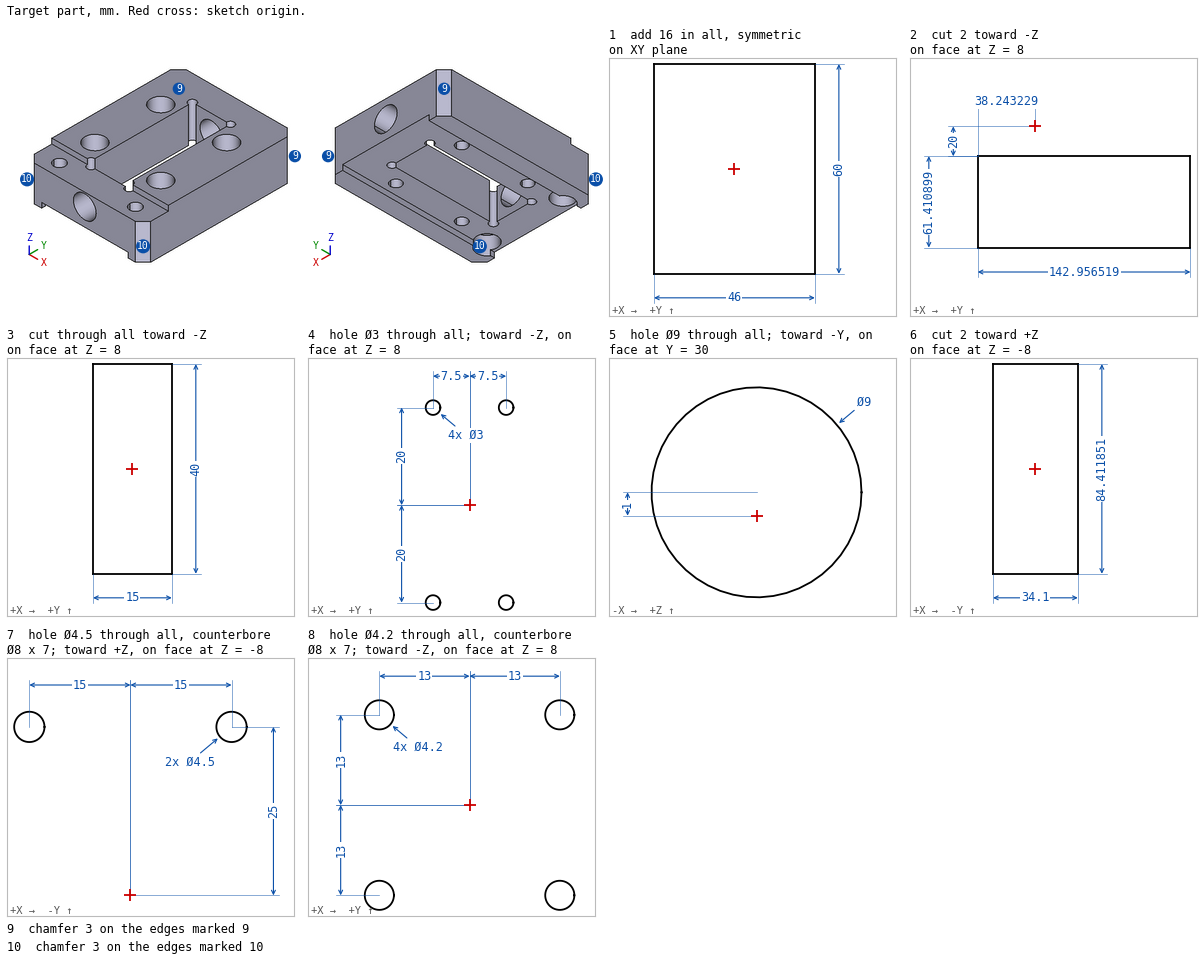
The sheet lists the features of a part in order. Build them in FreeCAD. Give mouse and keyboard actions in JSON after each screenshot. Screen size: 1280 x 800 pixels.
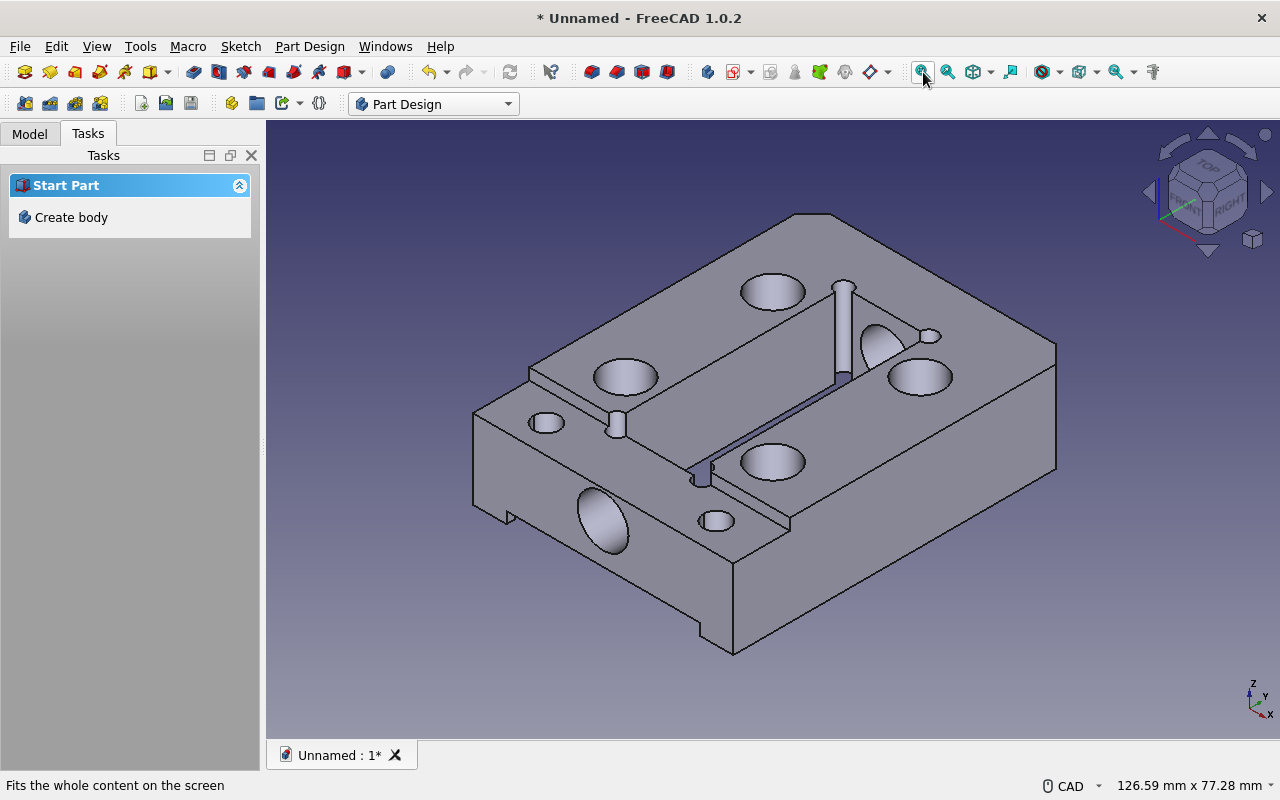
{"action": "left_click", "coordinate": [733, 608]}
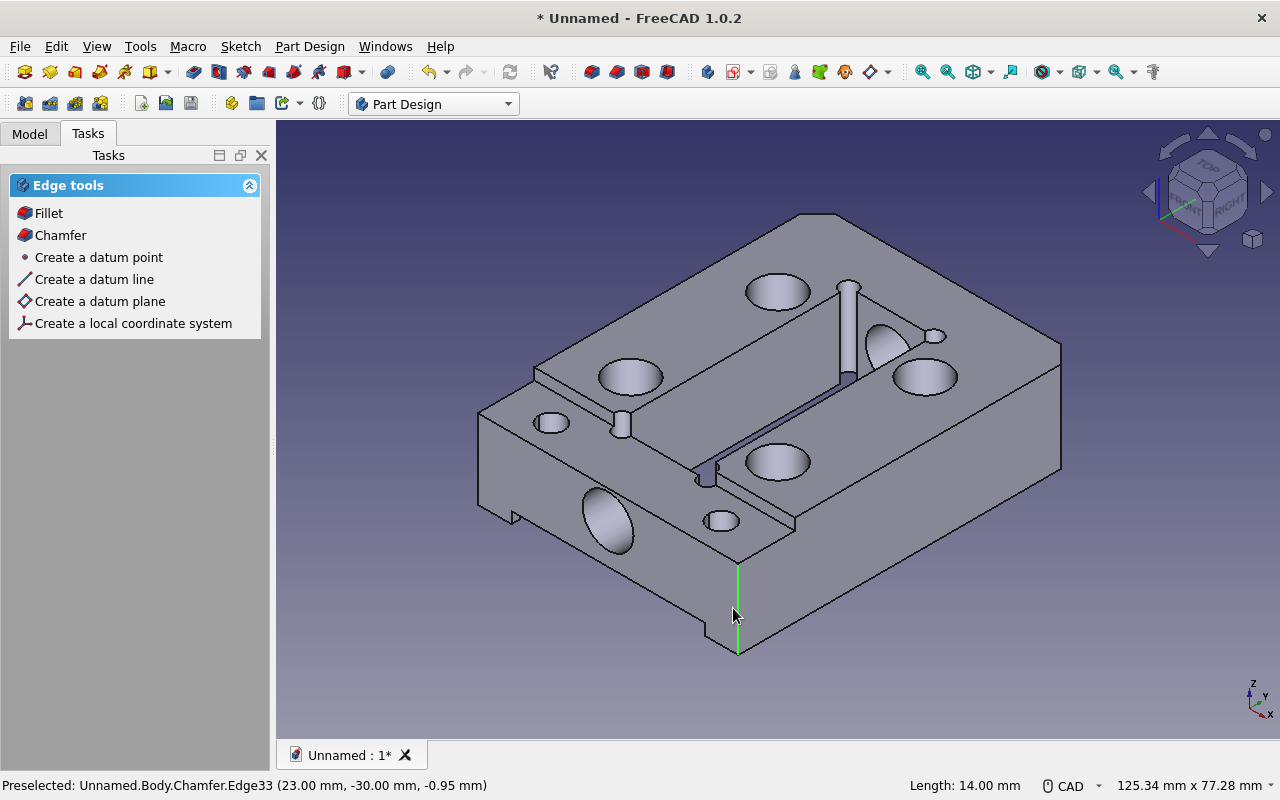
{"action": "key", "text": "2"}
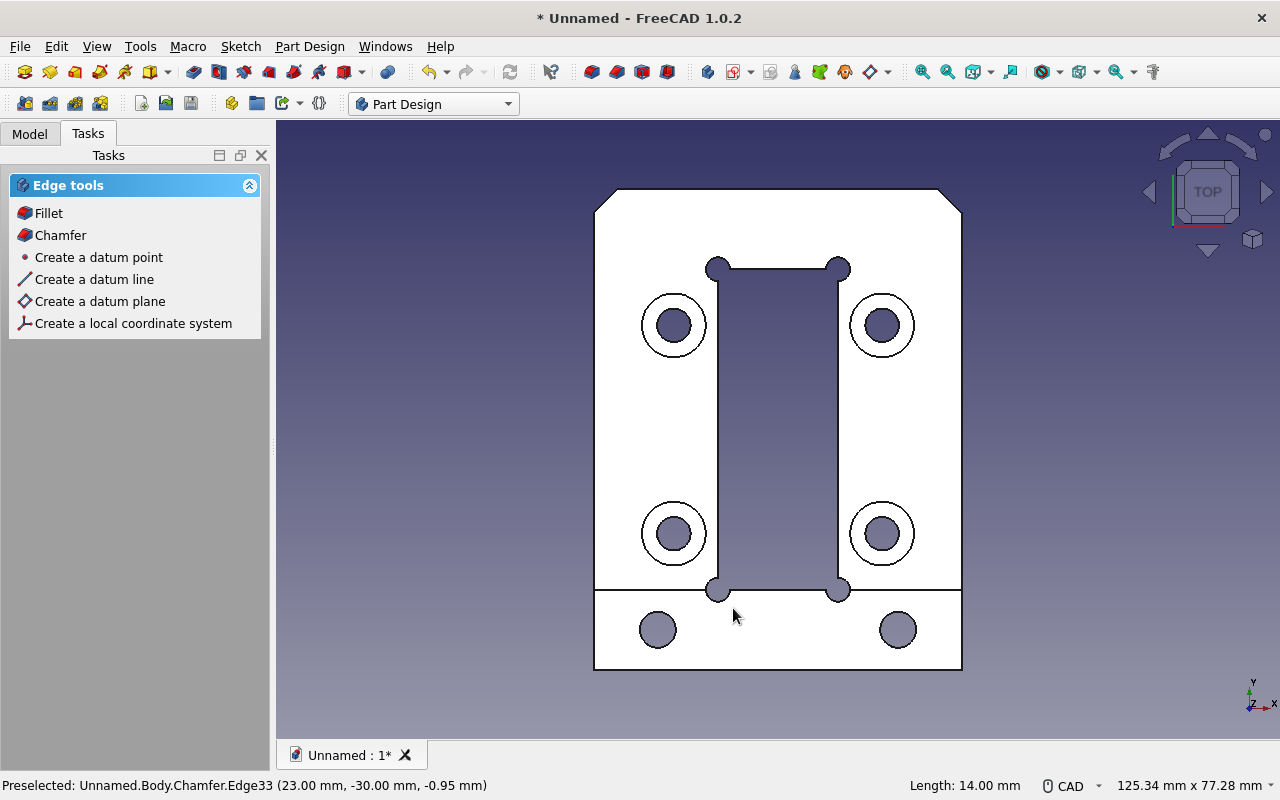
{"action": "key", "text": "1"}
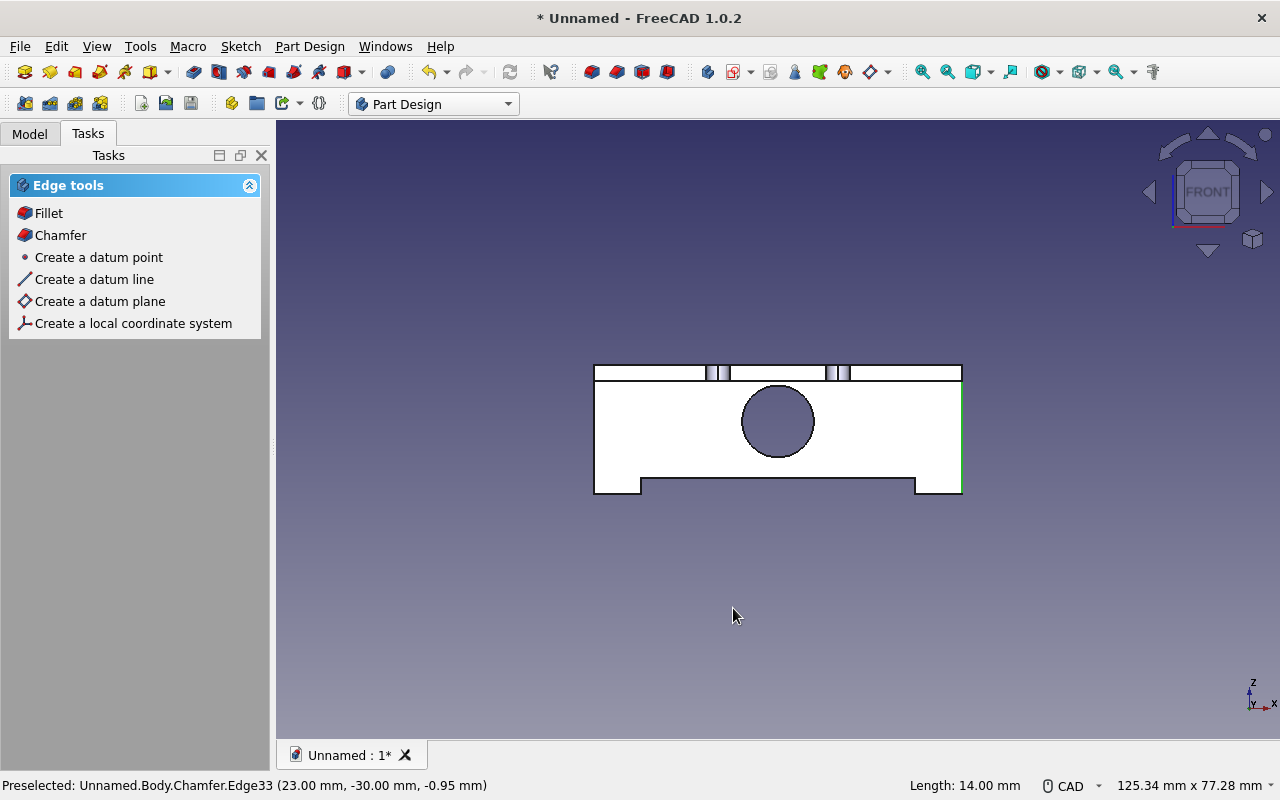
{"action": "left_click", "coordinate": [923, 72]}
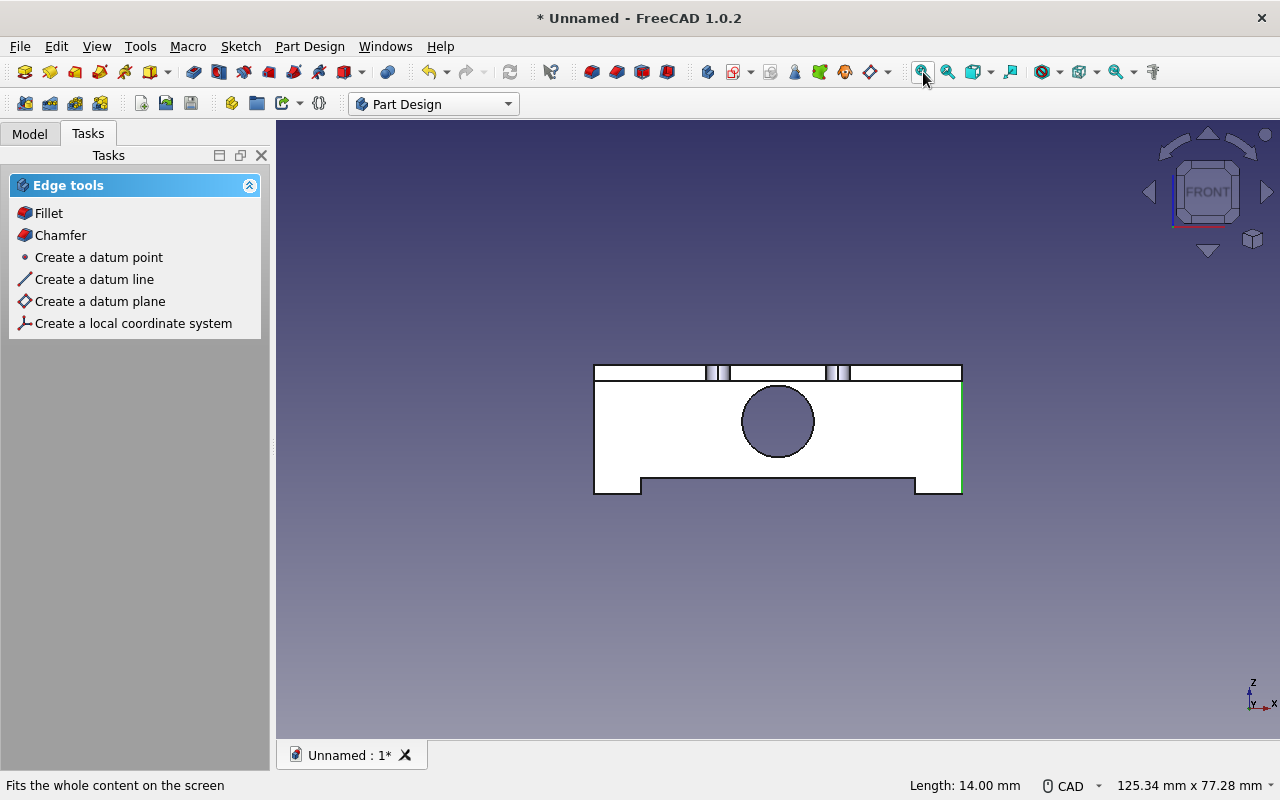
{"action": "left_click", "coordinate": [594, 437], "text": "ctrl"}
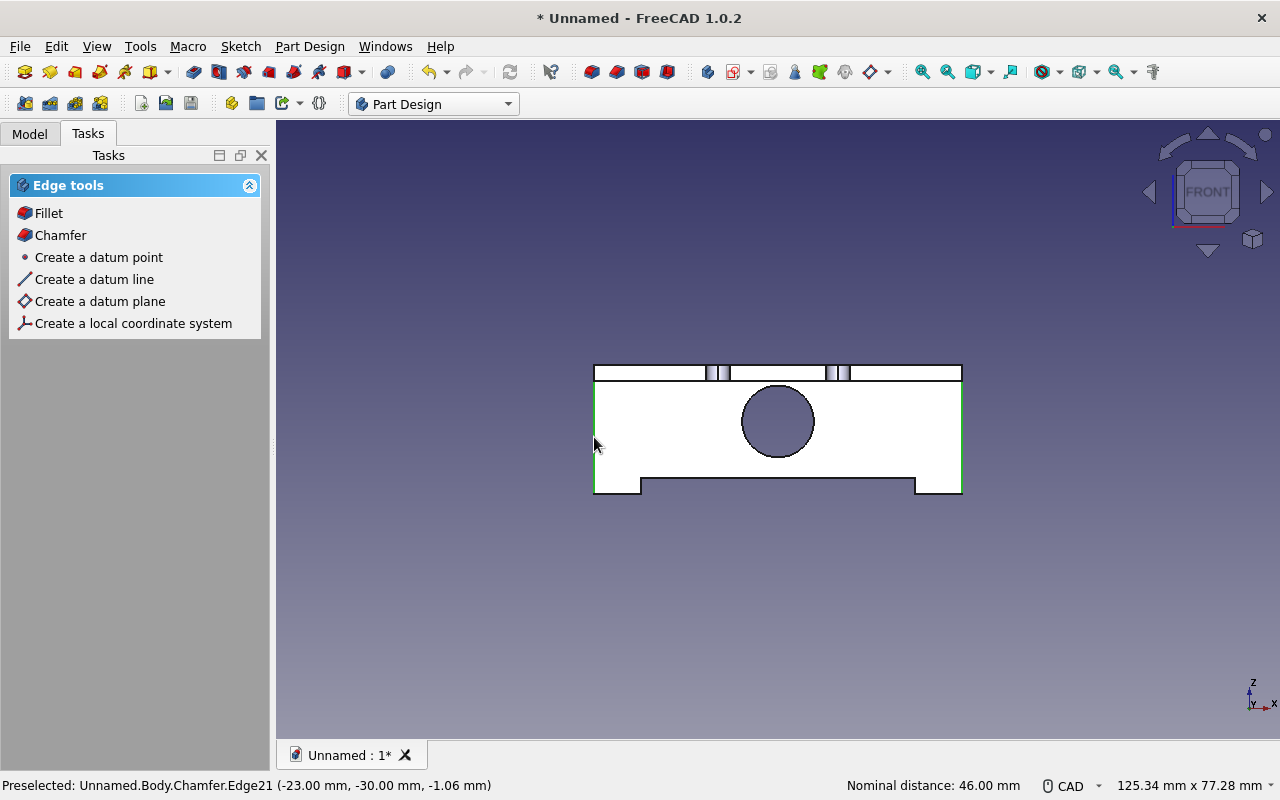
{"action": "left_click", "coordinate": [617, 72]}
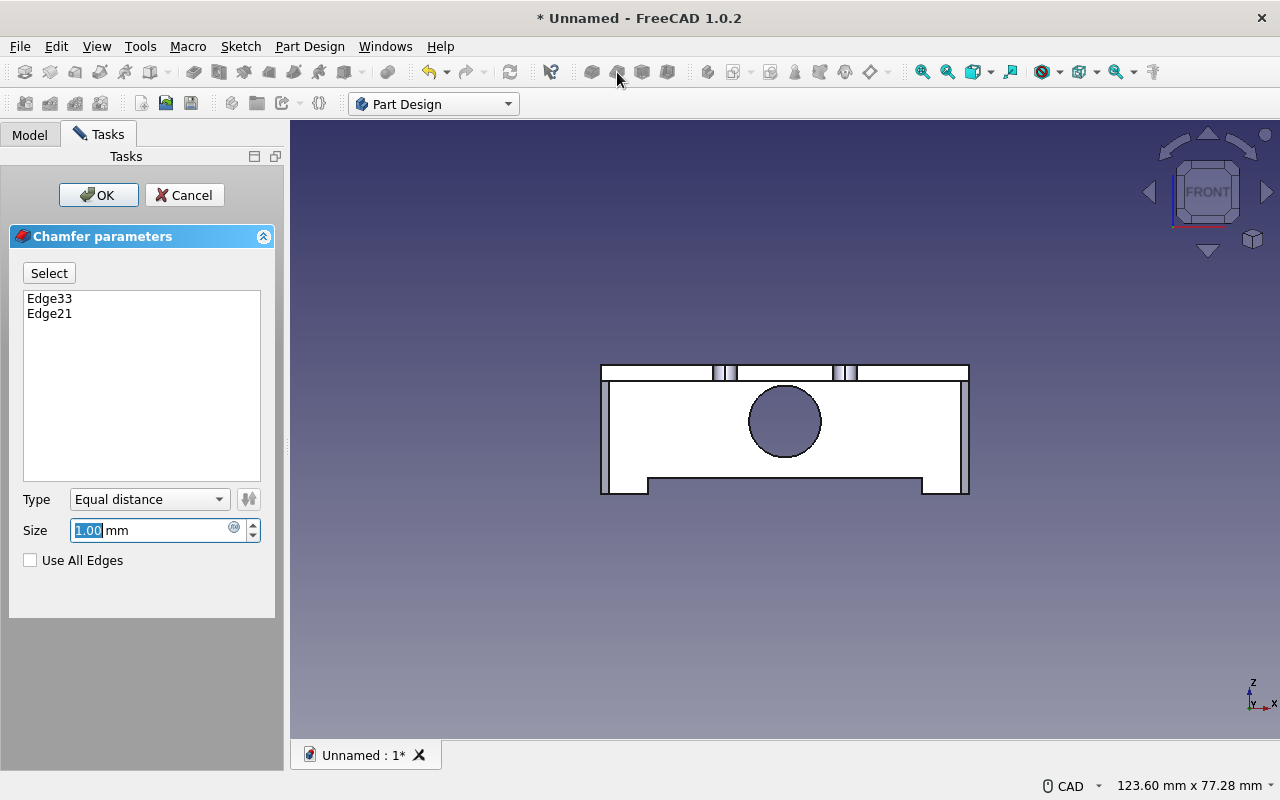
{"action": "type", "text": "3"}
{"action": "key", "text": "Tab"}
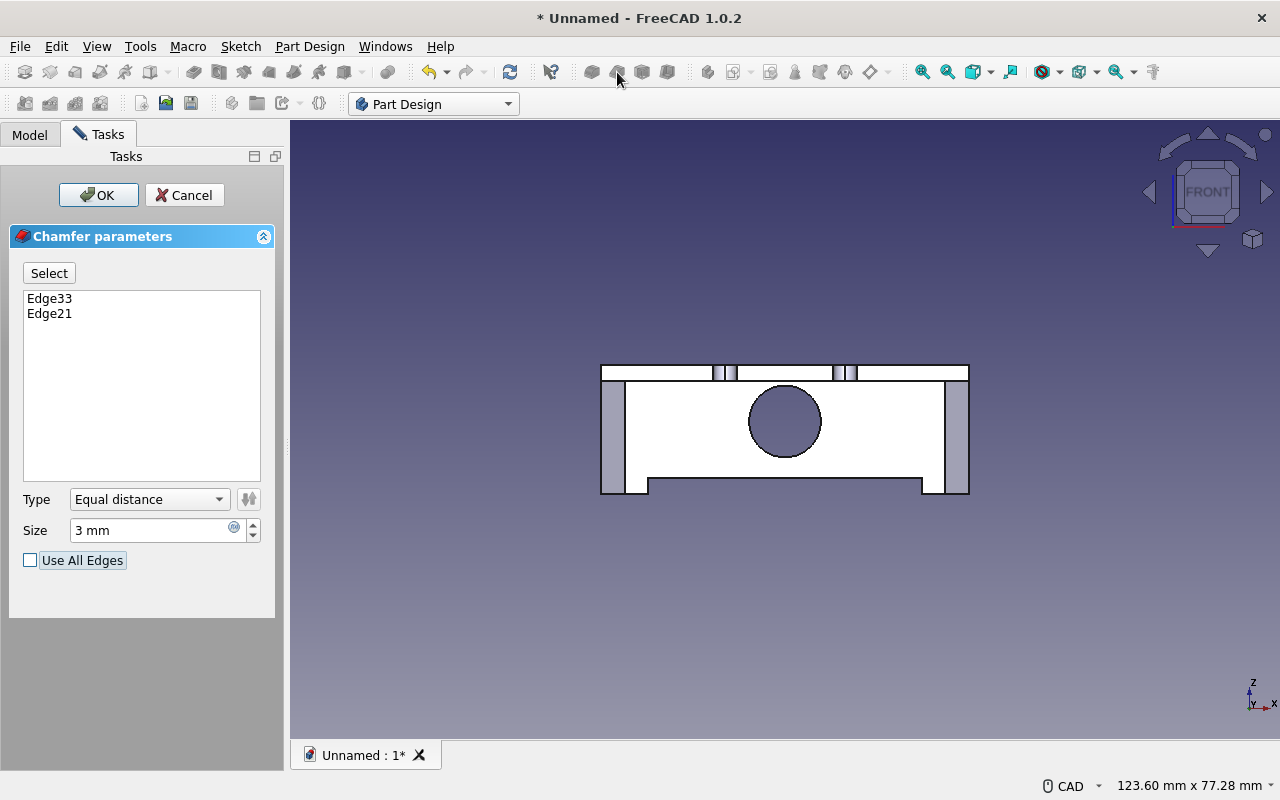
{"action": "left_click", "coordinate": [99, 195]}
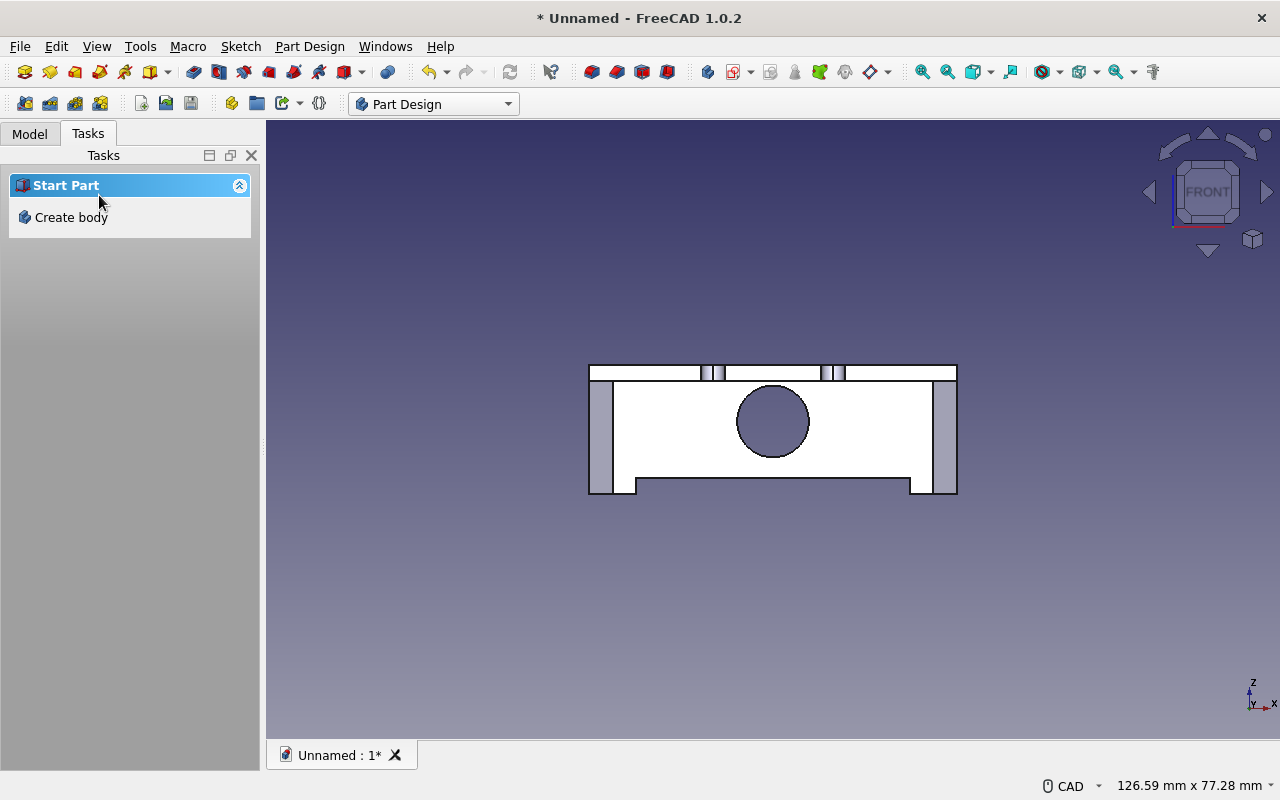
{"action": "key", "text": "0"}